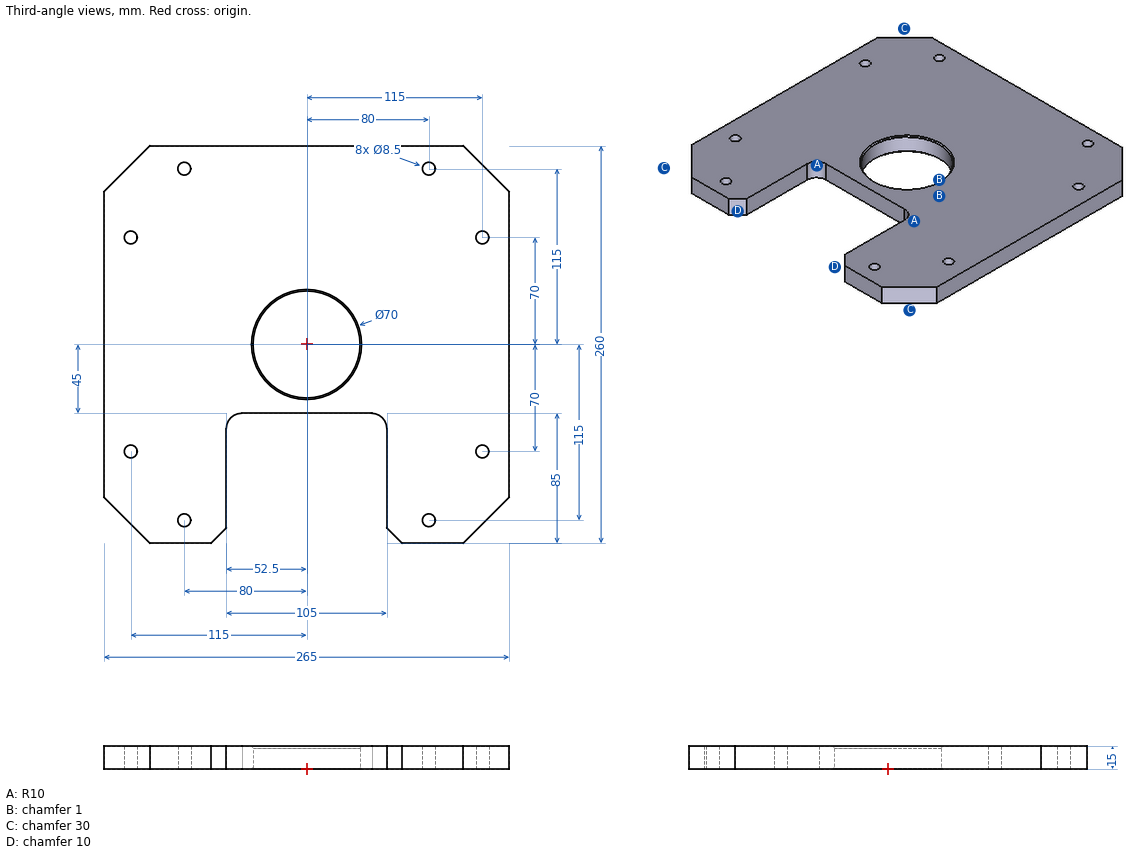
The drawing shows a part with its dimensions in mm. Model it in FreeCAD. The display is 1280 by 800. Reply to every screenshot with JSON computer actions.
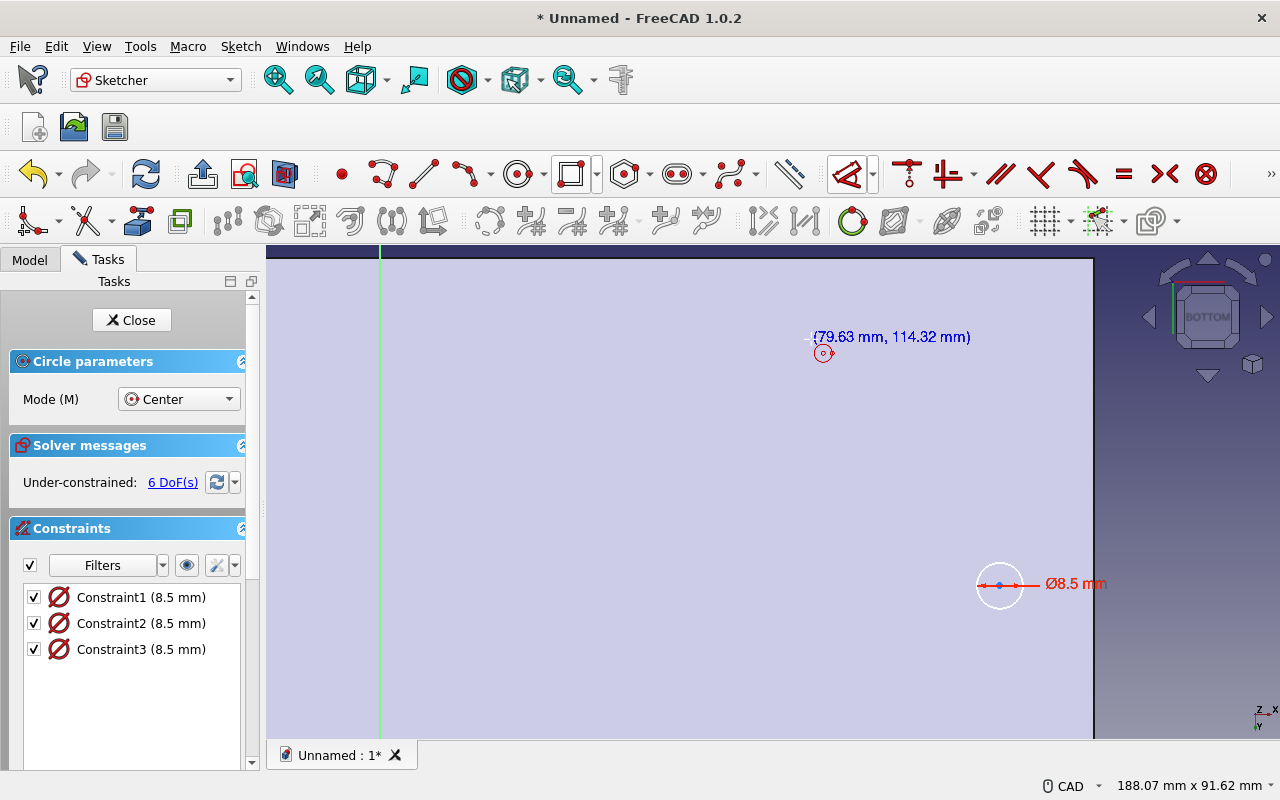
{"action": "scroll", "coordinate": [811, 339], "scroll_direction": "down", "scroll_amount": 7}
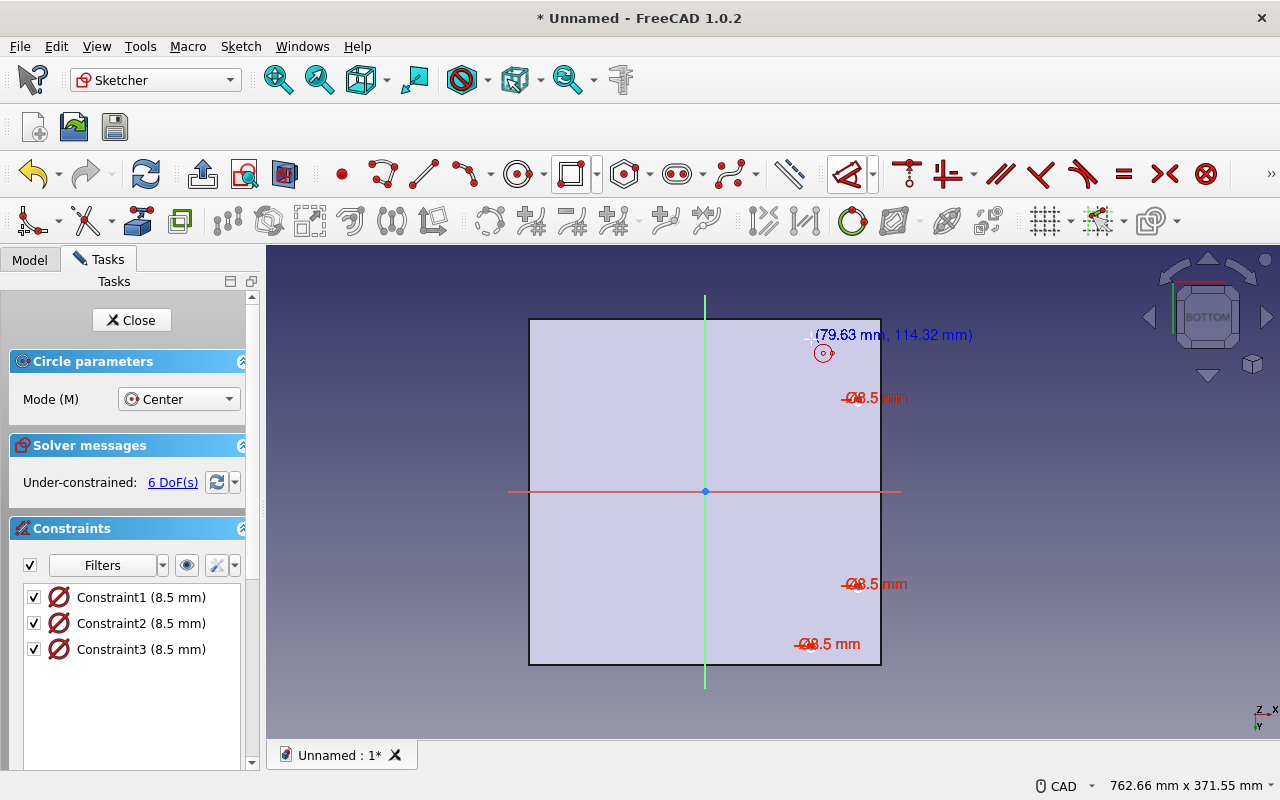
{"action": "left_click", "coordinate": [811, 339]}
{"action": "mouse_move", "coordinate": [815, 335]}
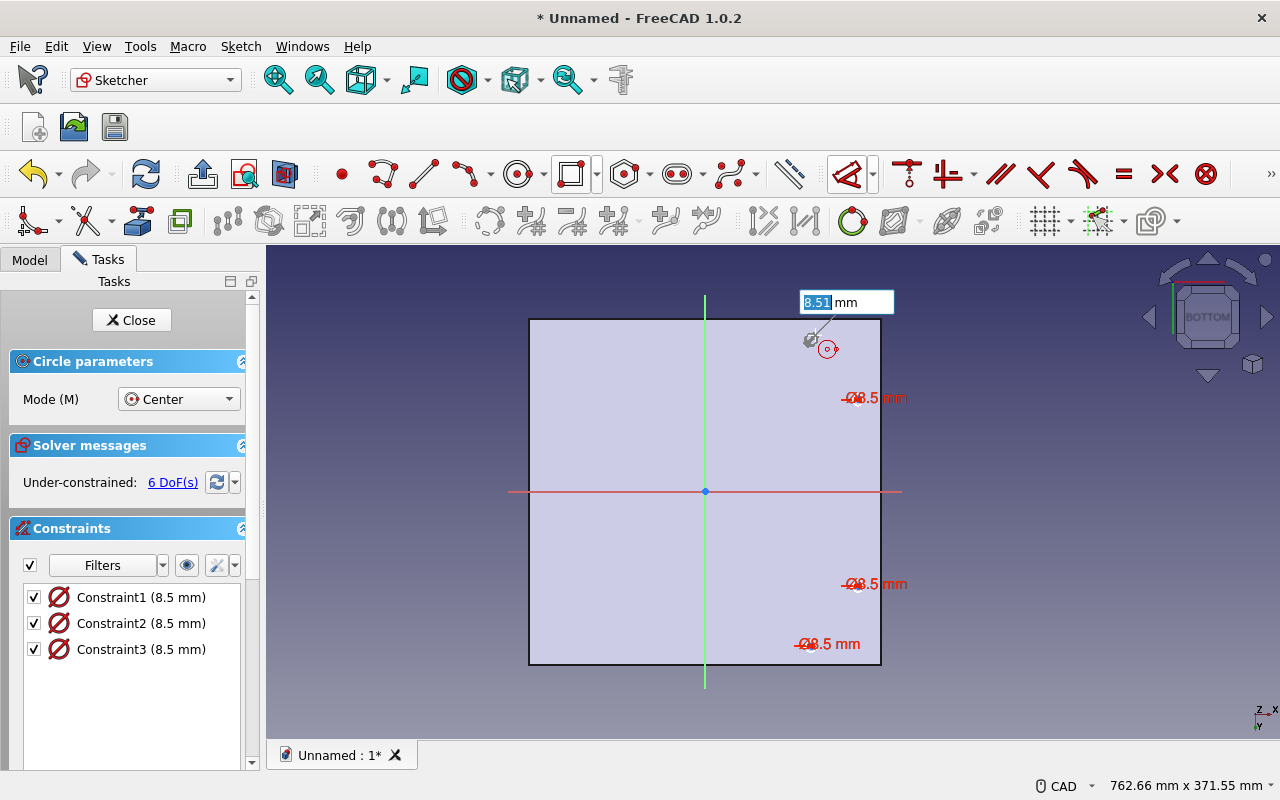
{"action": "type", "text": "8.5"}
{"action": "key", "text": "Return"}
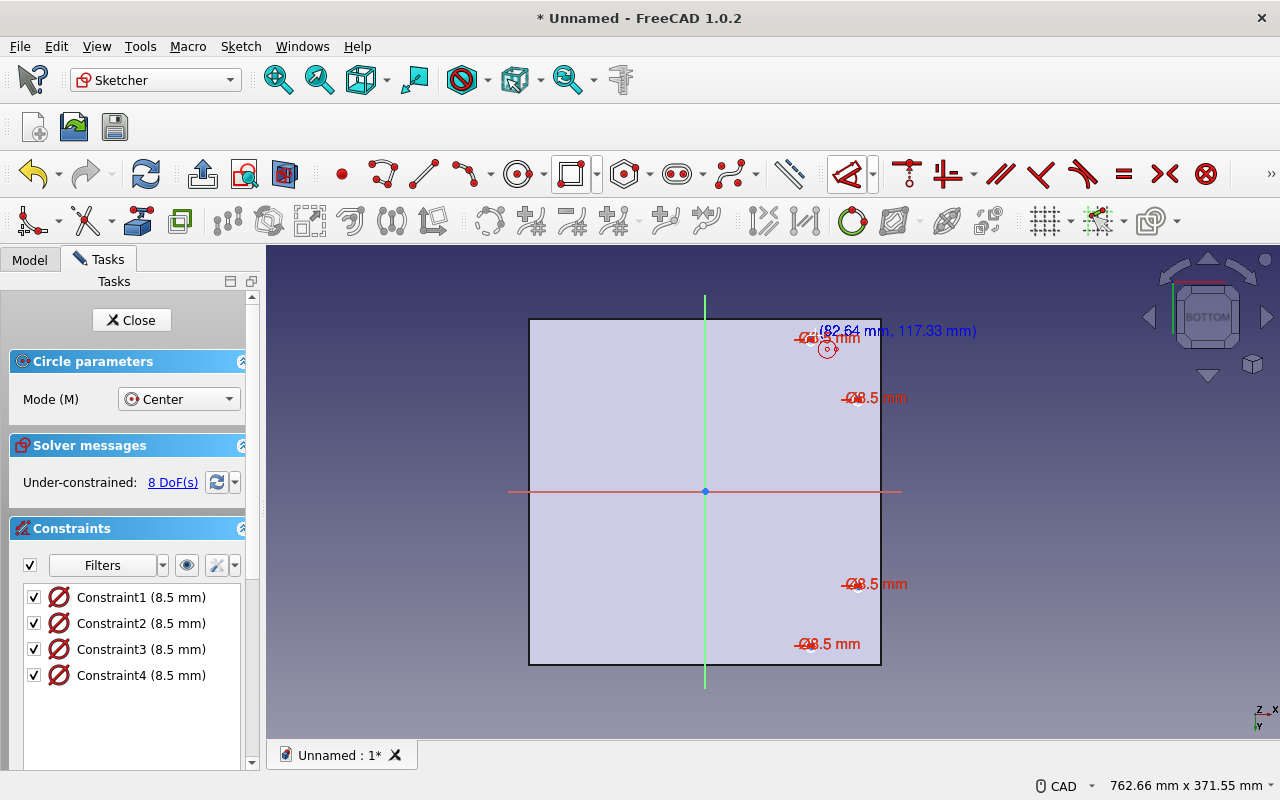
{"action": "scroll", "coordinate": [599, 339], "scroll_direction": "up", "scroll_amount": 7}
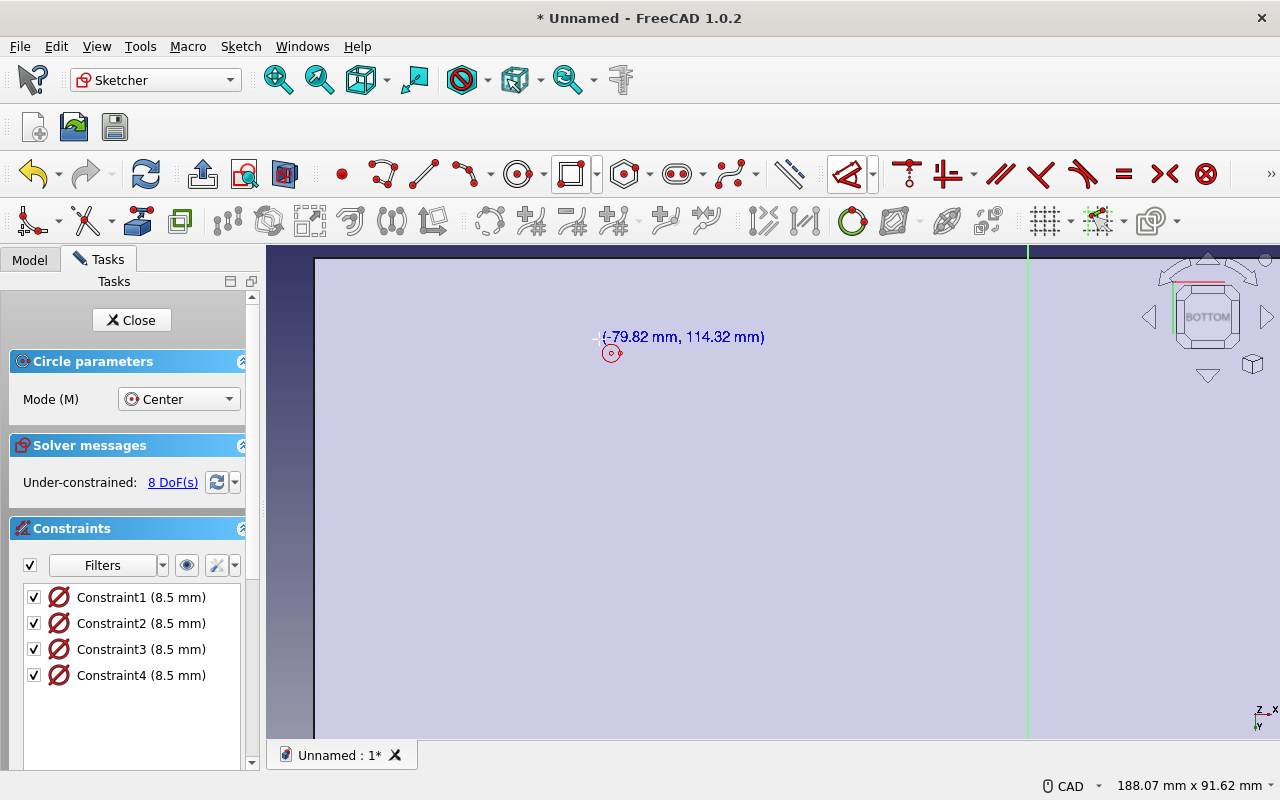
{"action": "scroll", "coordinate": [598, 339], "scroll_direction": "down", "scroll_amount": 7}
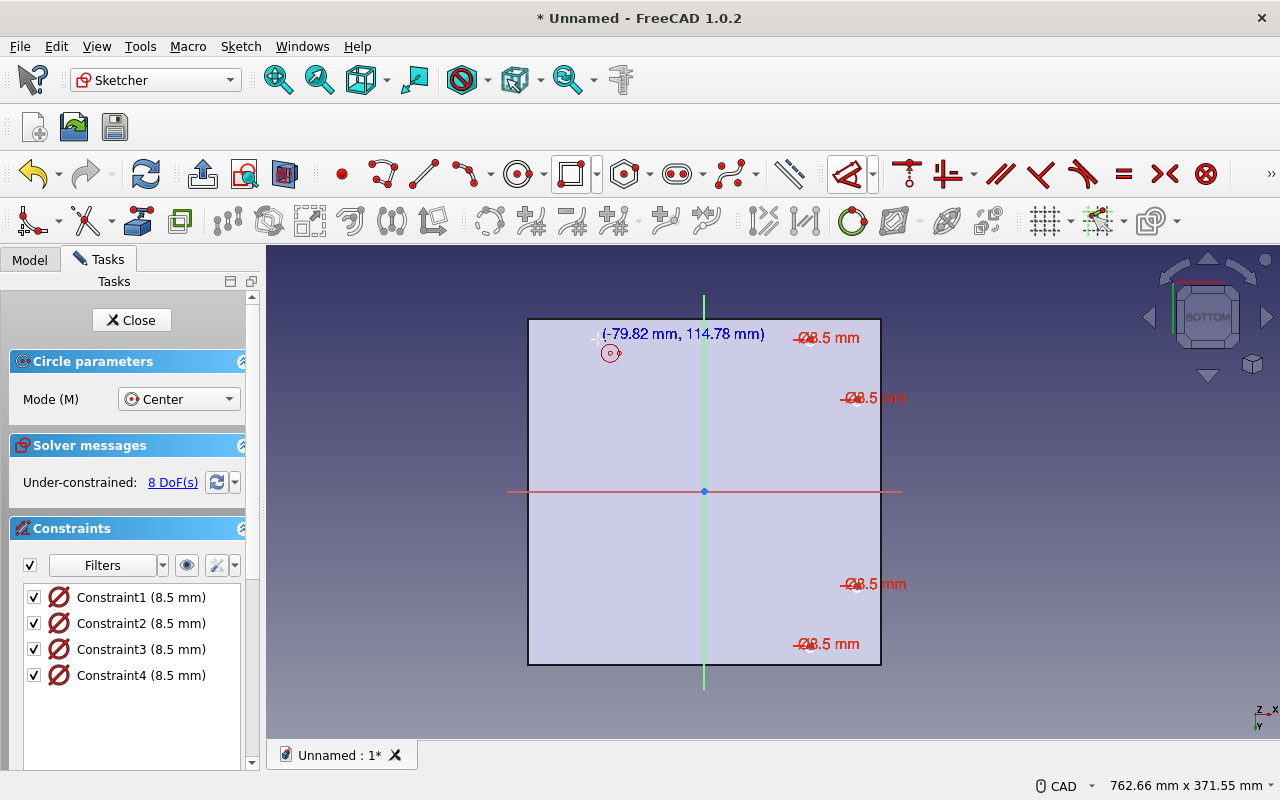
{"action": "left_click", "coordinate": [598, 339]}
{"action": "mouse_move", "coordinate": [602, 335]}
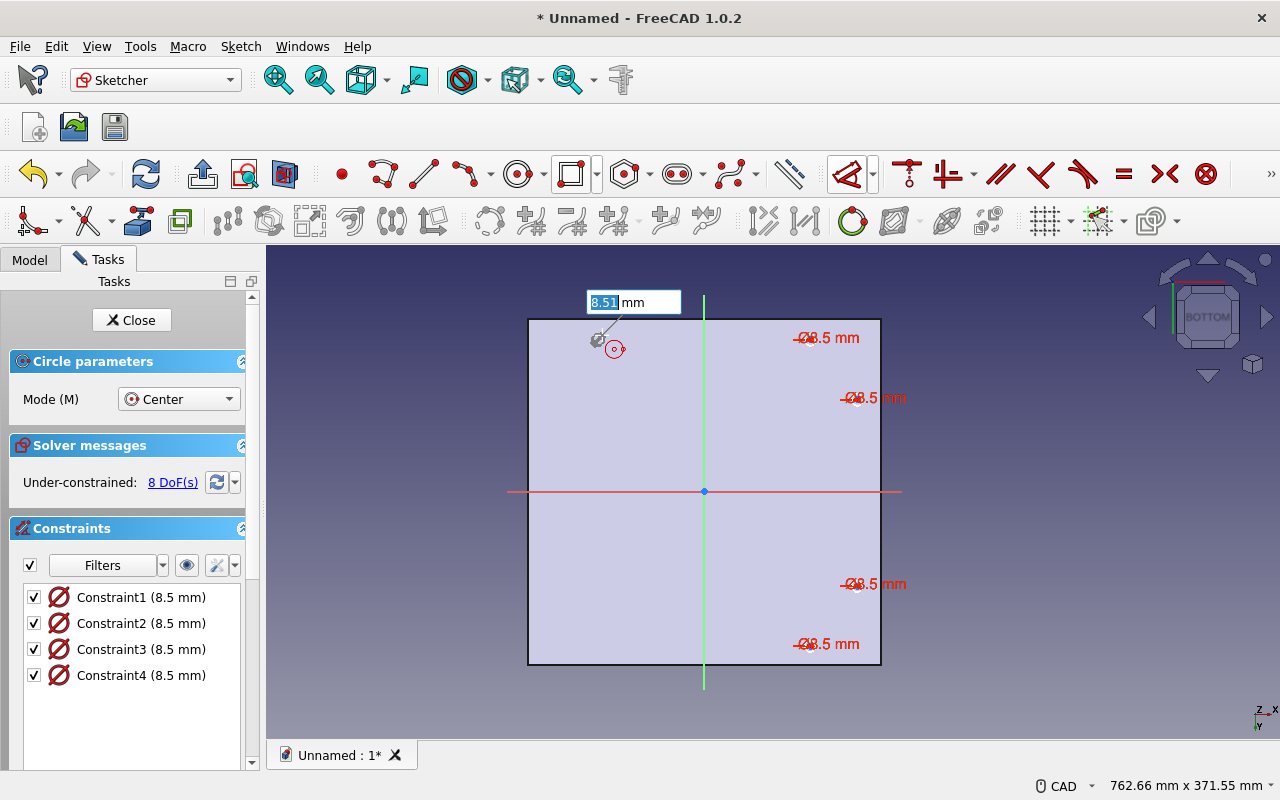
{"action": "type", "text": "8.5"}
{"action": "key", "text": "Return"}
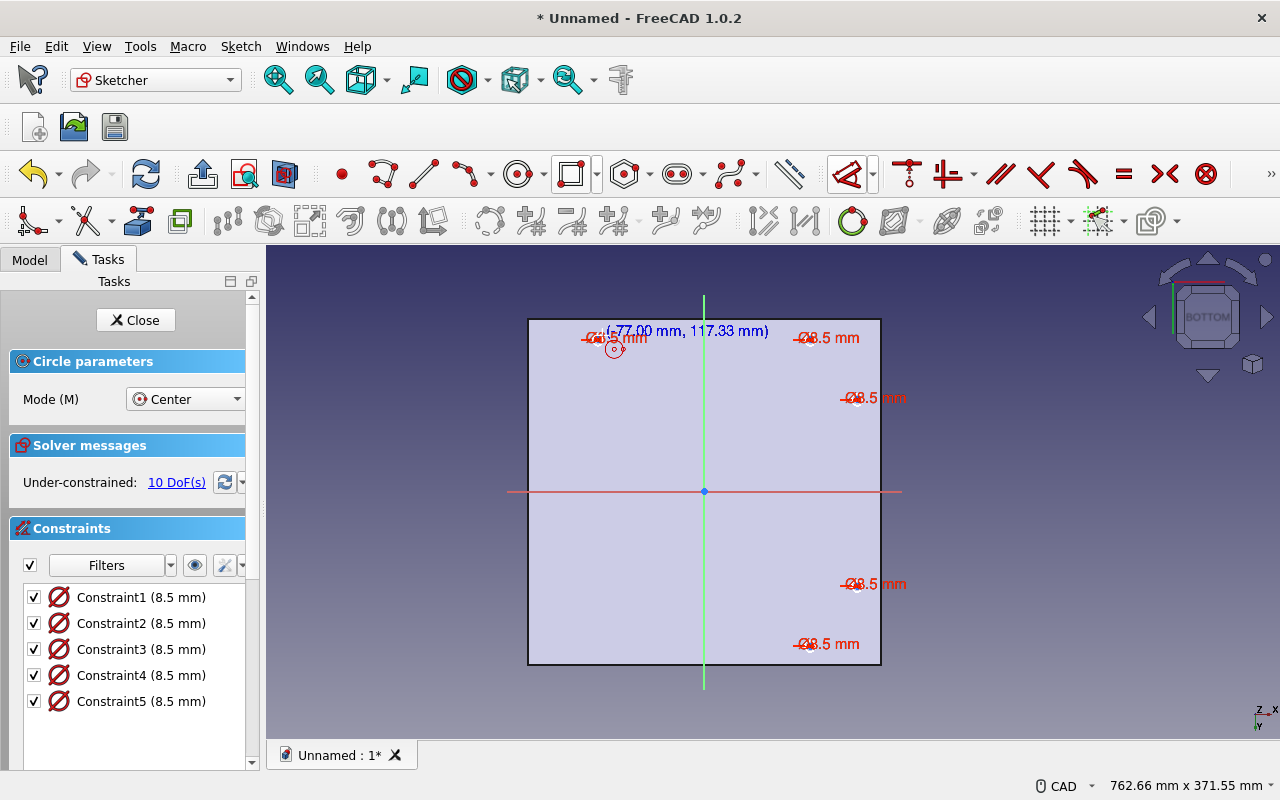
{"action": "scroll", "coordinate": [551, 399], "scroll_direction": "up", "scroll_amount": 7}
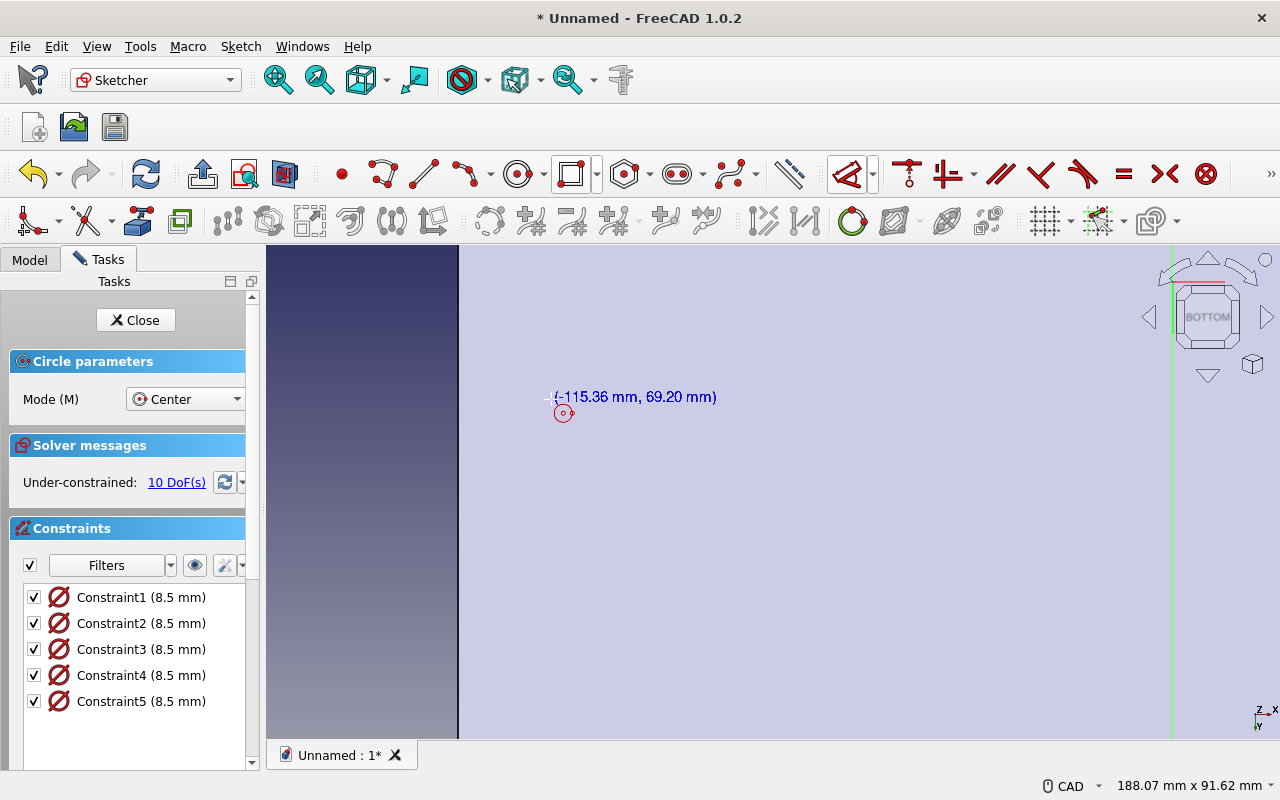
{"action": "scroll", "coordinate": [551, 399], "scroll_direction": "down", "scroll_amount": 7}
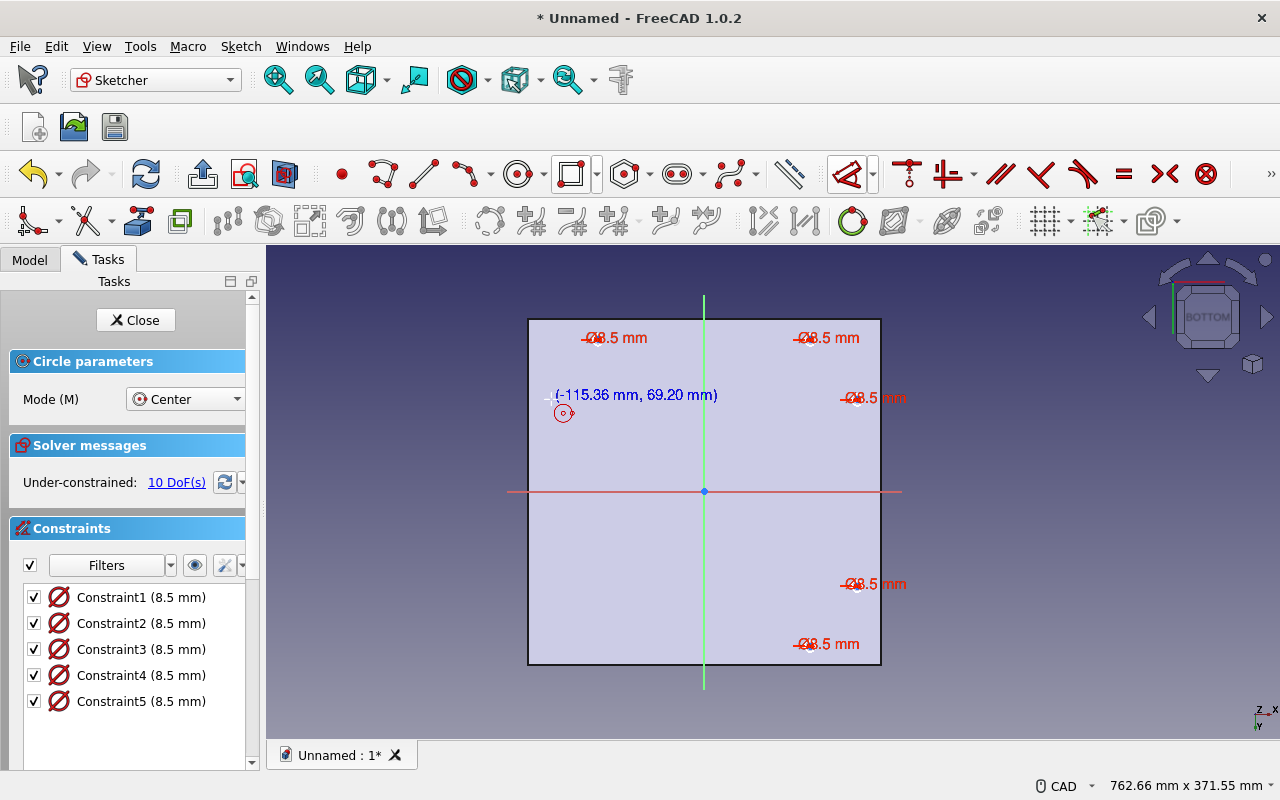
{"action": "left_click", "coordinate": [551, 399]}
{"action": "mouse_move", "coordinate": [555, 395]}